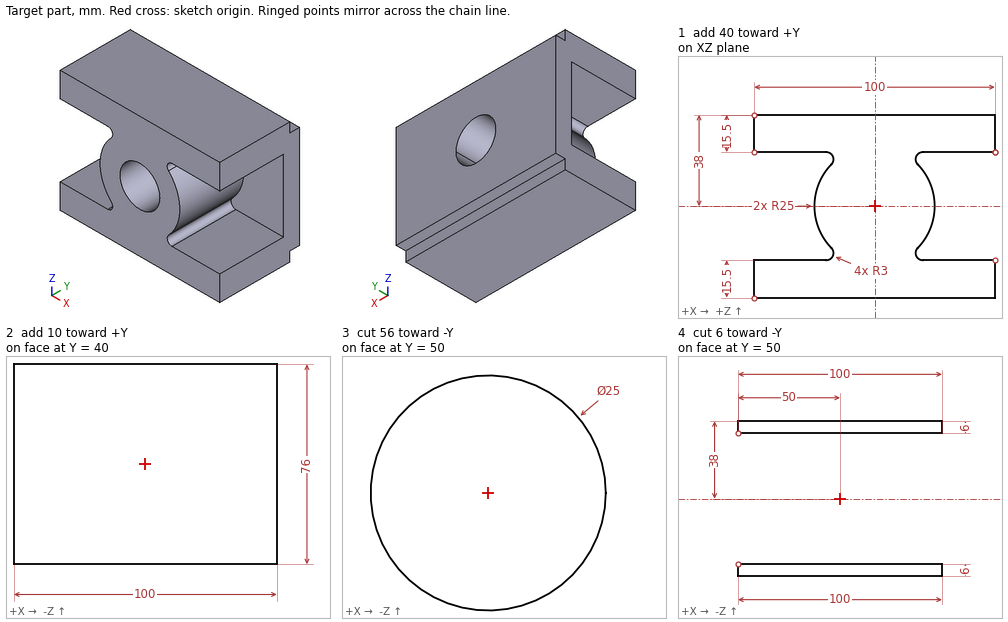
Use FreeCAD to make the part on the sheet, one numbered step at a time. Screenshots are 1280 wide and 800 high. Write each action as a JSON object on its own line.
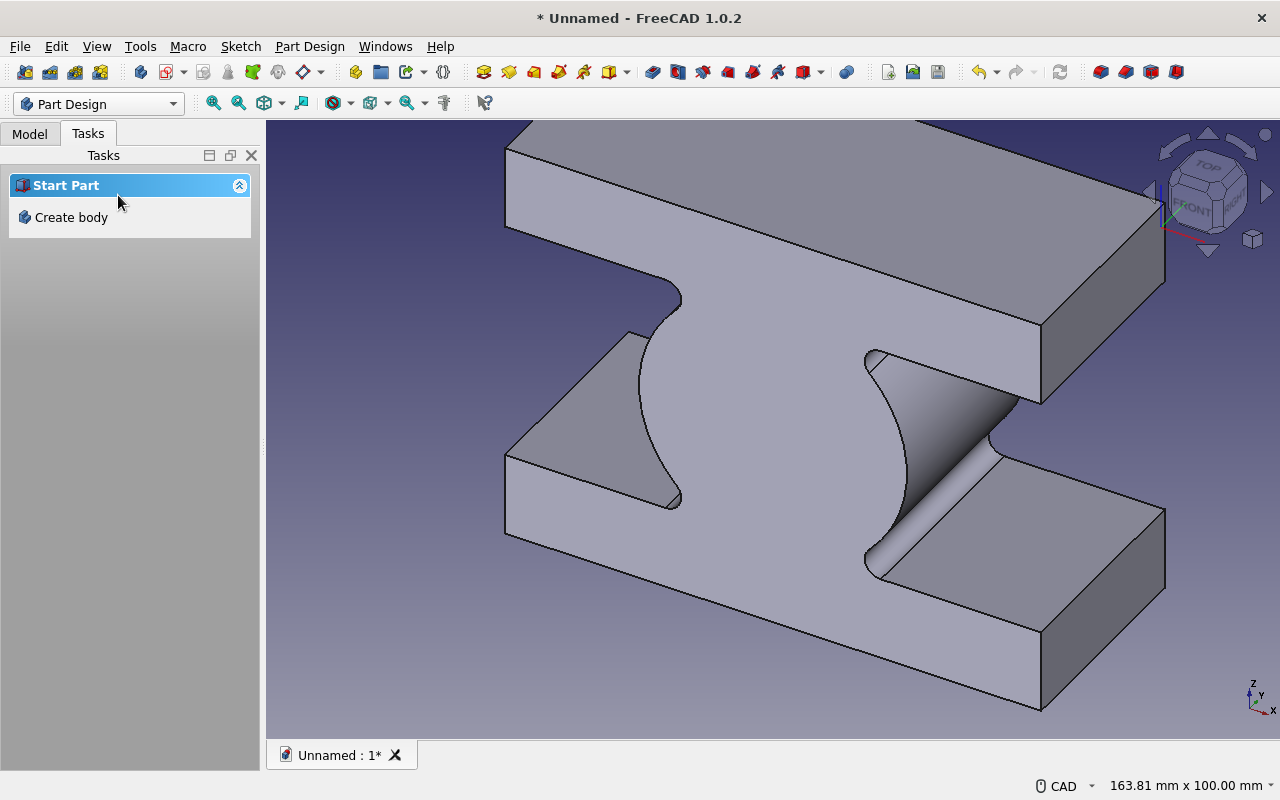
{"action": "key", "text": "v f"}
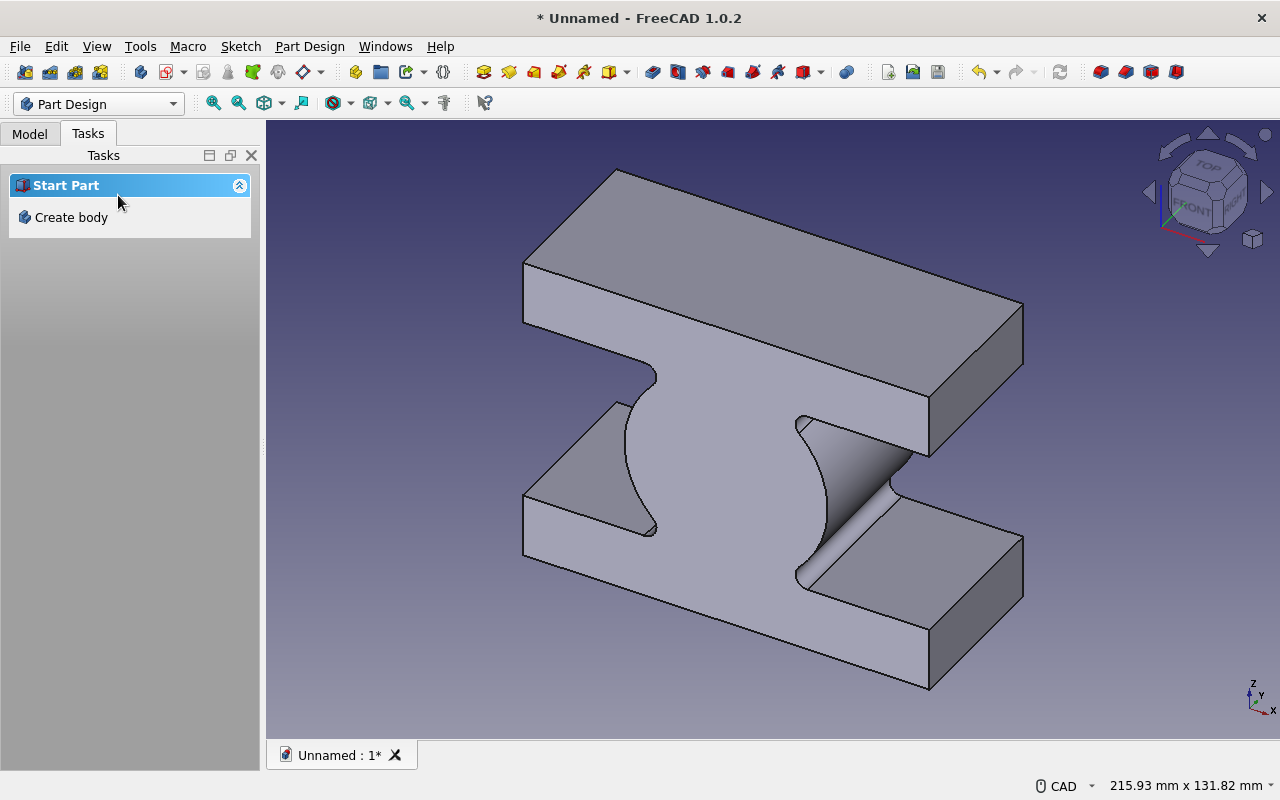
{"action": "key", "text": "4"}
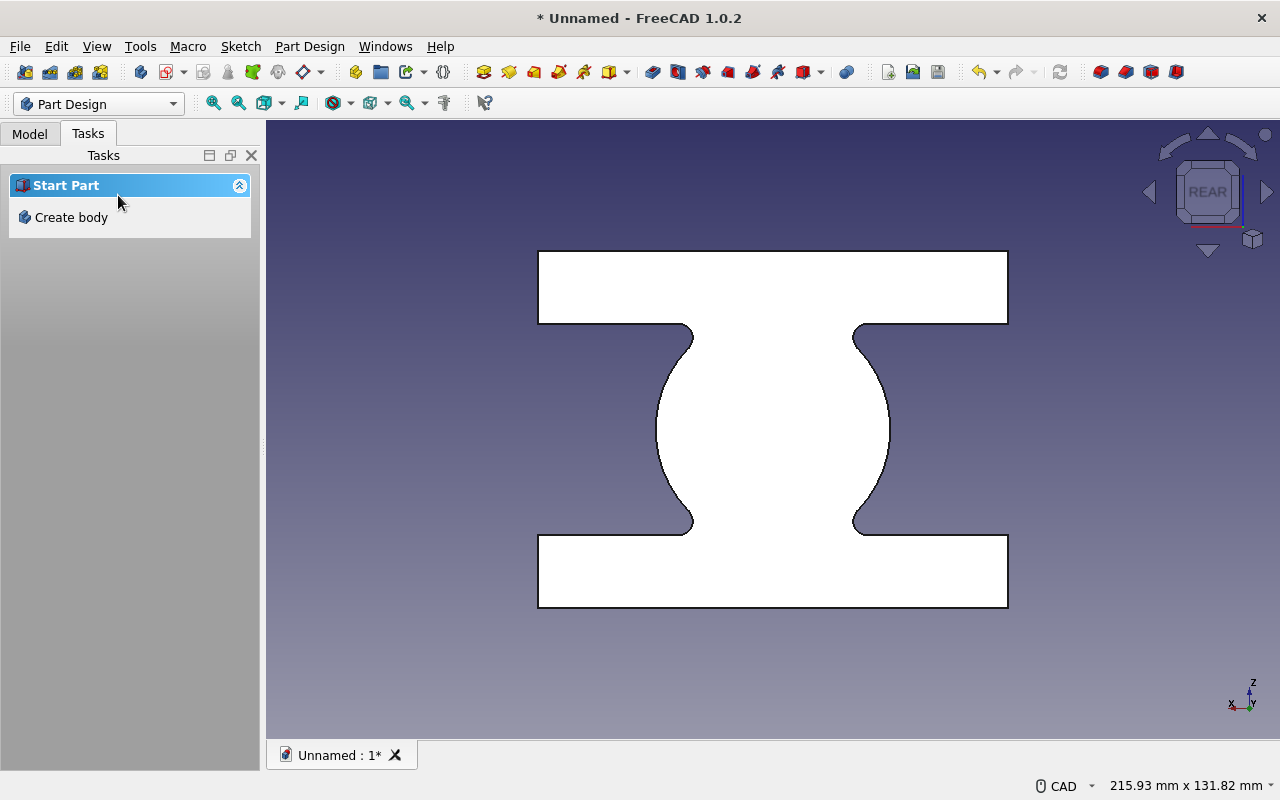
{"action": "left_click", "coordinate": [773, 428]}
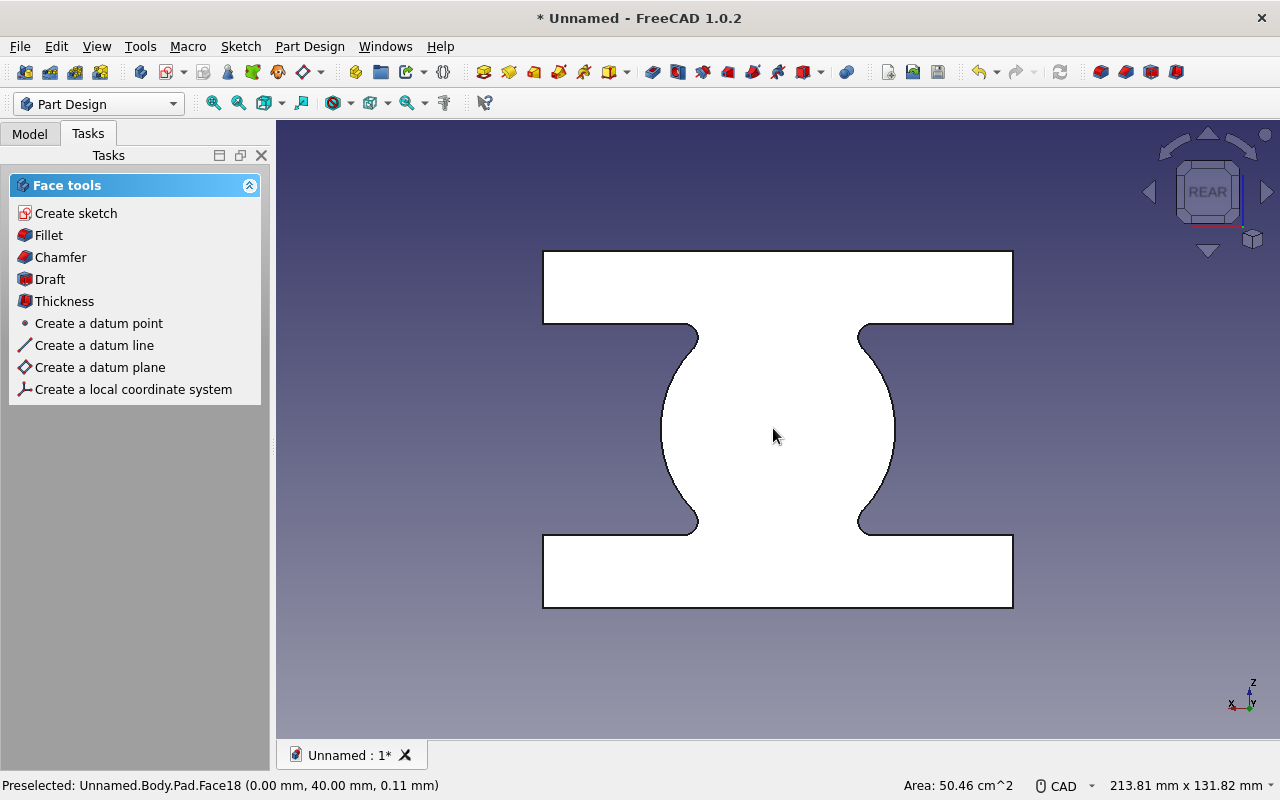
{"action": "left_click", "coordinate": [166, 72]}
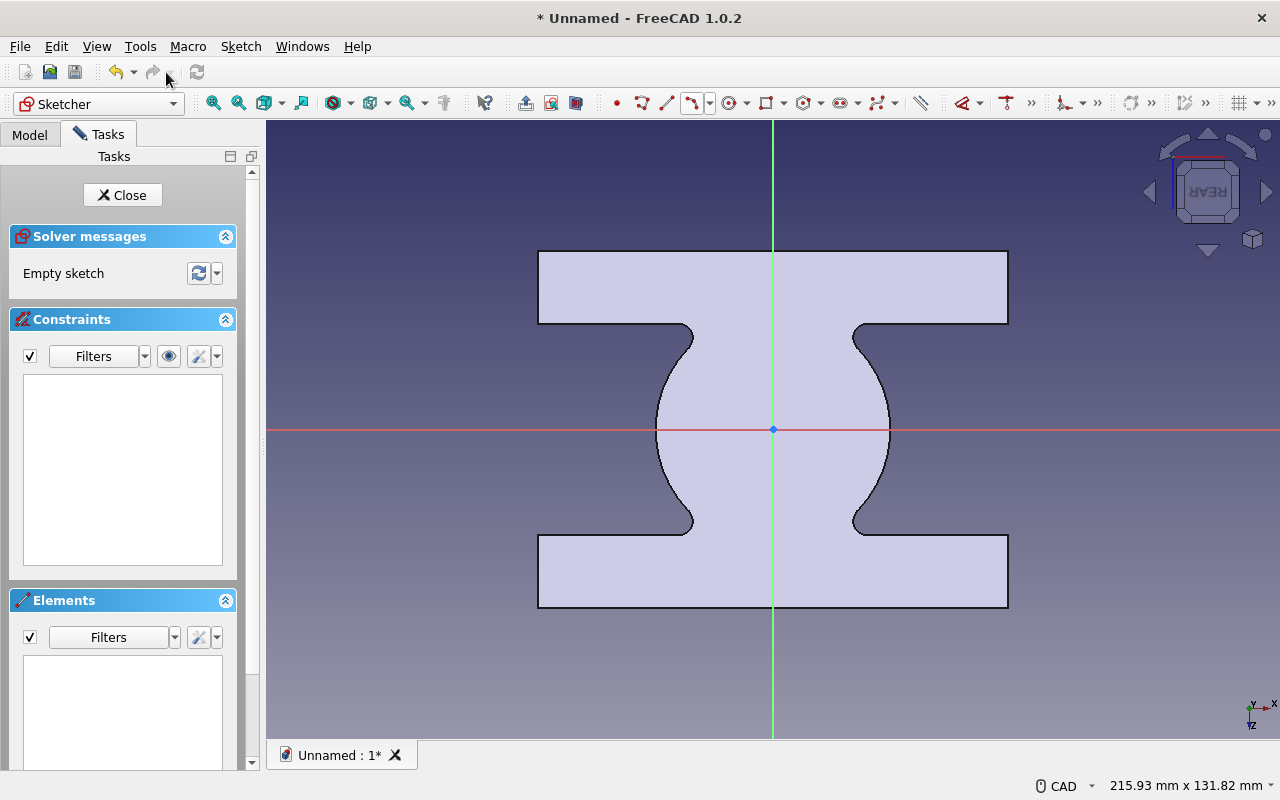
{"action": "left_click", "coordinate": [784, 104]}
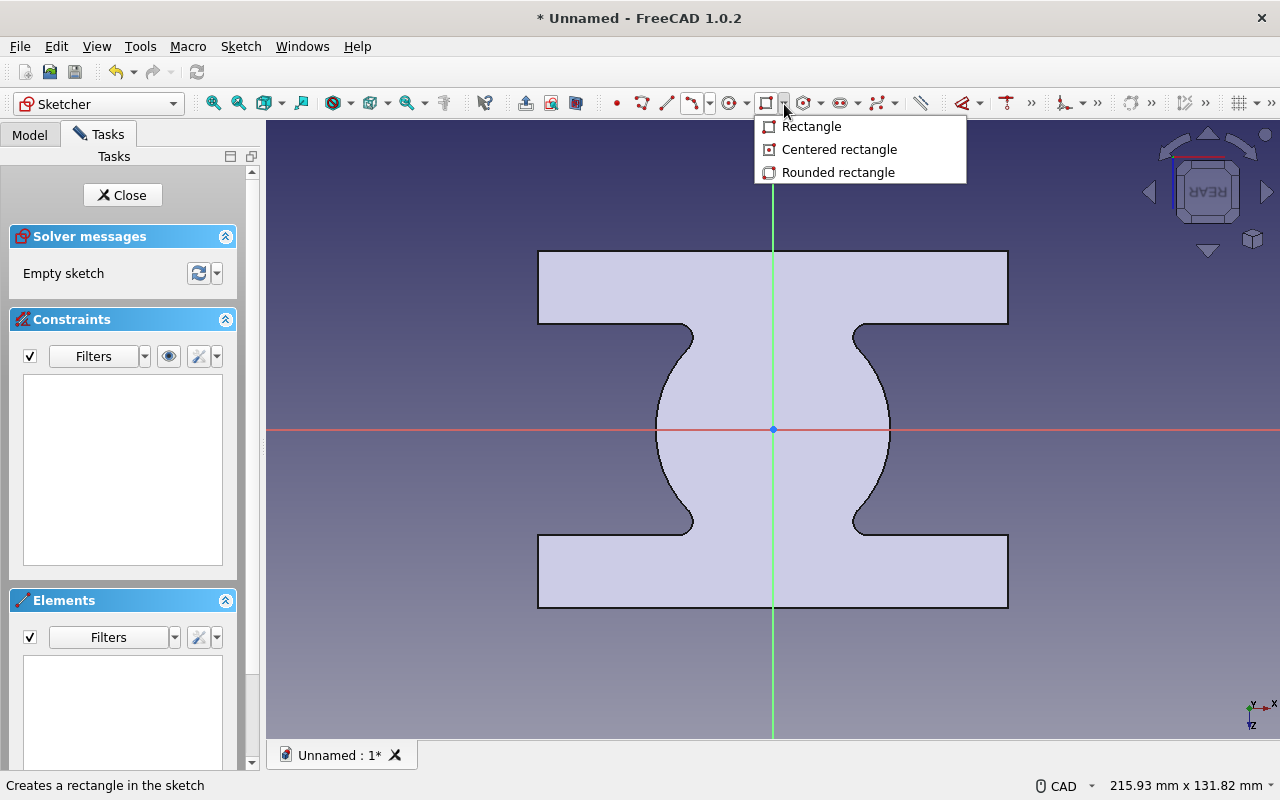
{"action": "left_click", "coordinate": [860, 150]}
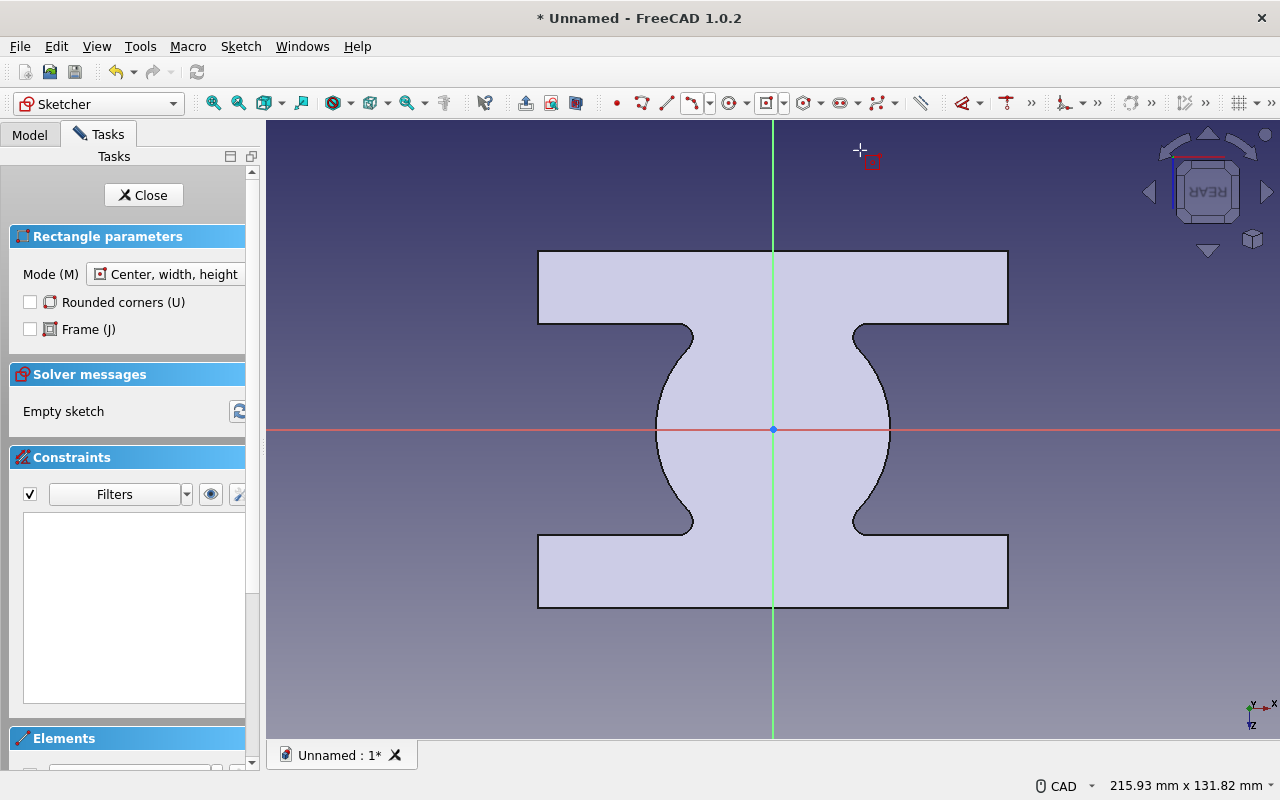
{"action": "left_click", "coordinate": [773, 430]}
{"action": "mouse_move", "coordinate": [1008, 251]}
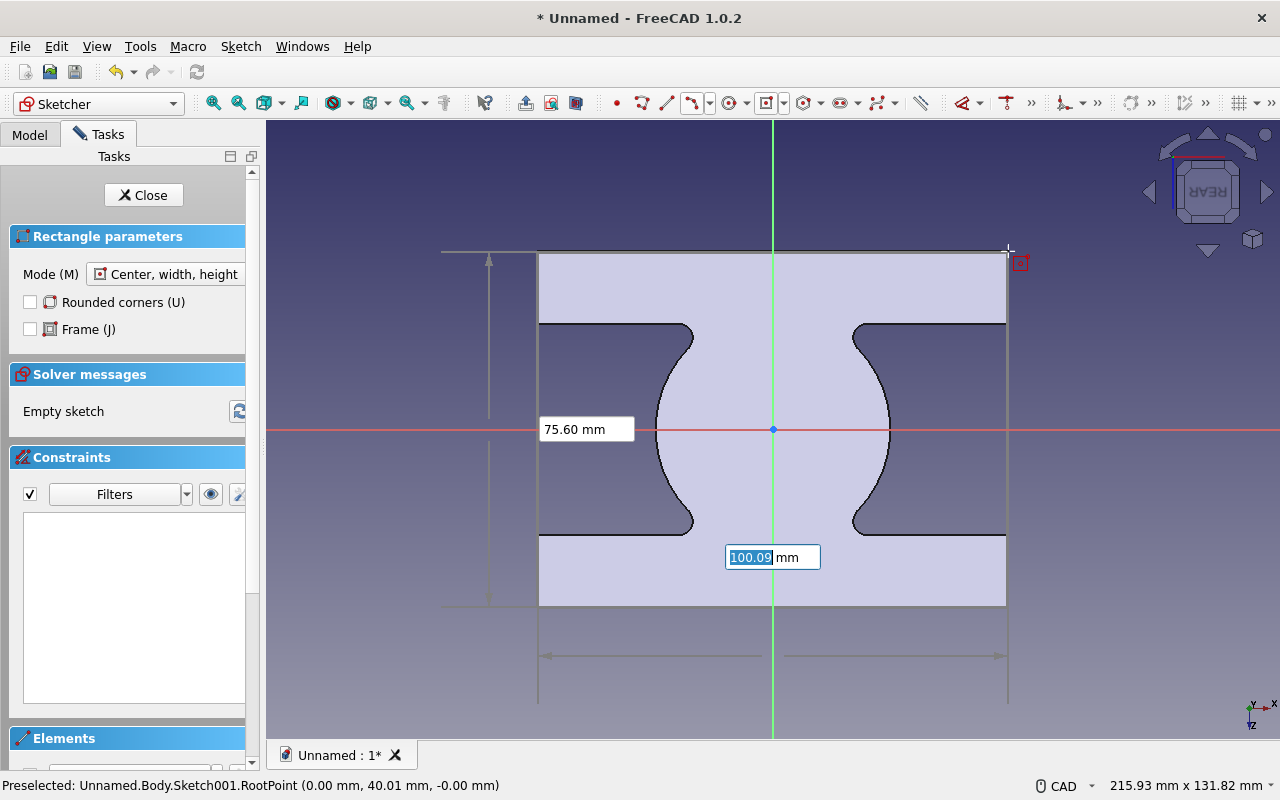
{"action": "type", "text": "100"}
{"action": "key", "text": "Tab"}
{"action": "type", "text": "76"}
{"action": "key", "text": "Return"}
{"action": "key", "text": "Escape"}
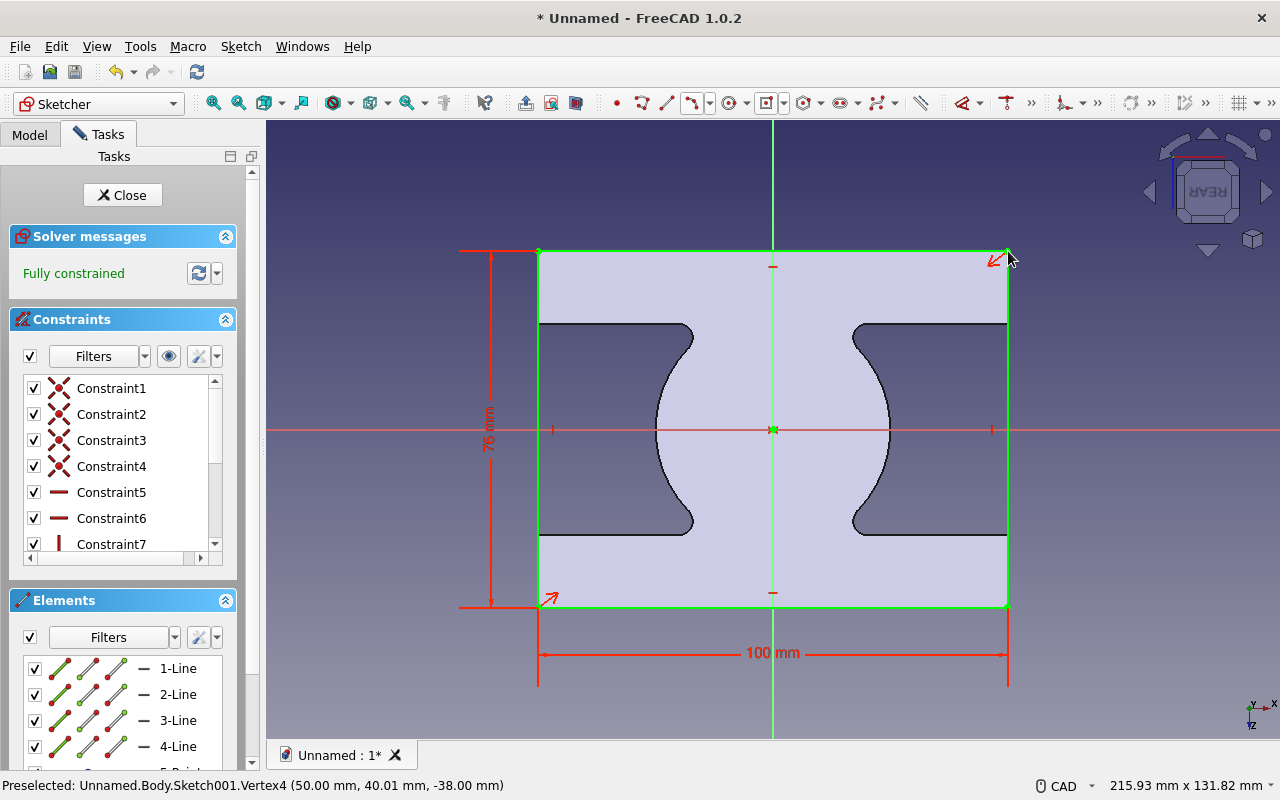
{"action": "left_click", "coordinate": [123, 195]}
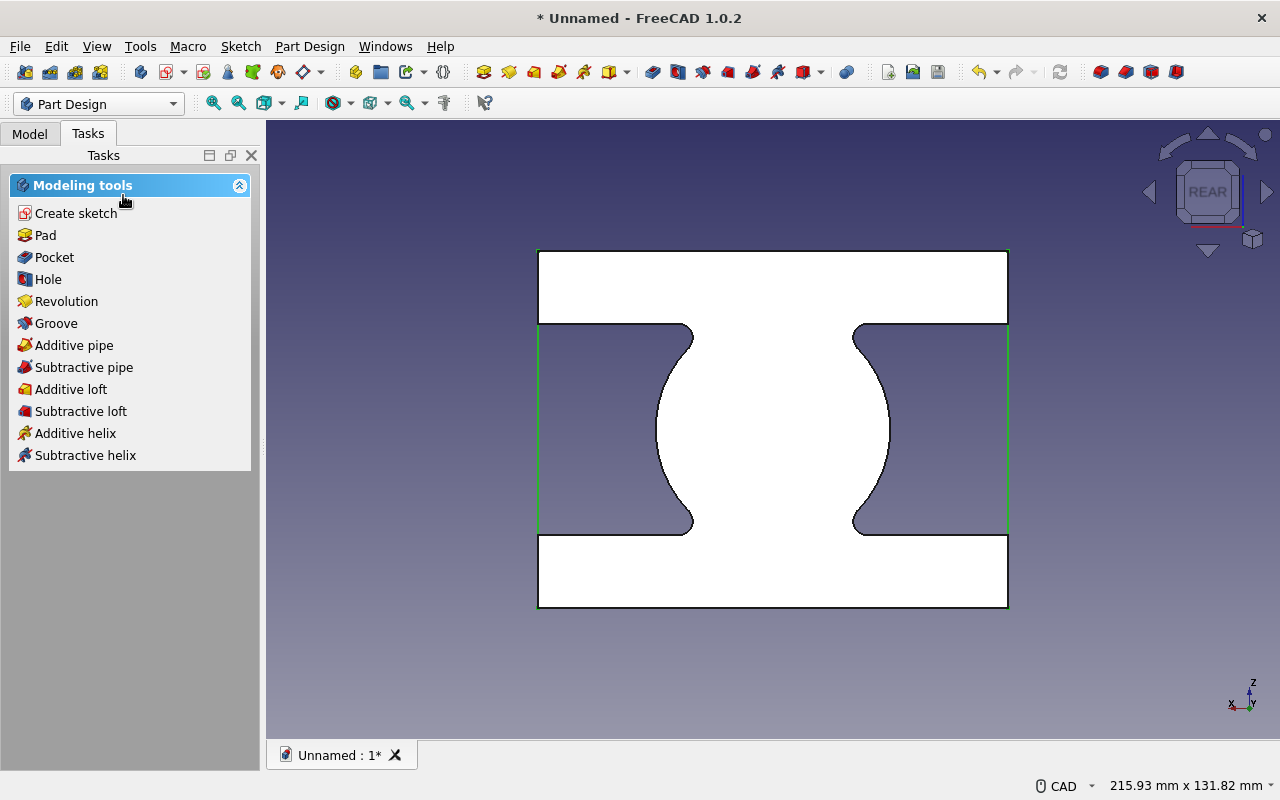
{"action": "left_click", "coordinate": [484, 72]}